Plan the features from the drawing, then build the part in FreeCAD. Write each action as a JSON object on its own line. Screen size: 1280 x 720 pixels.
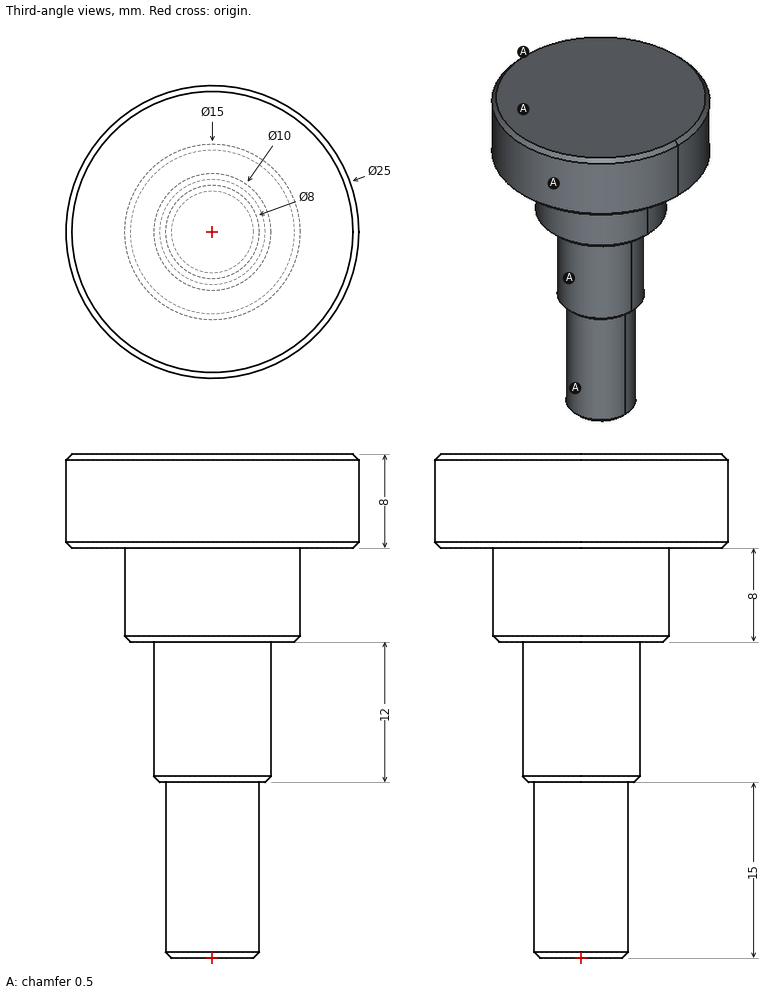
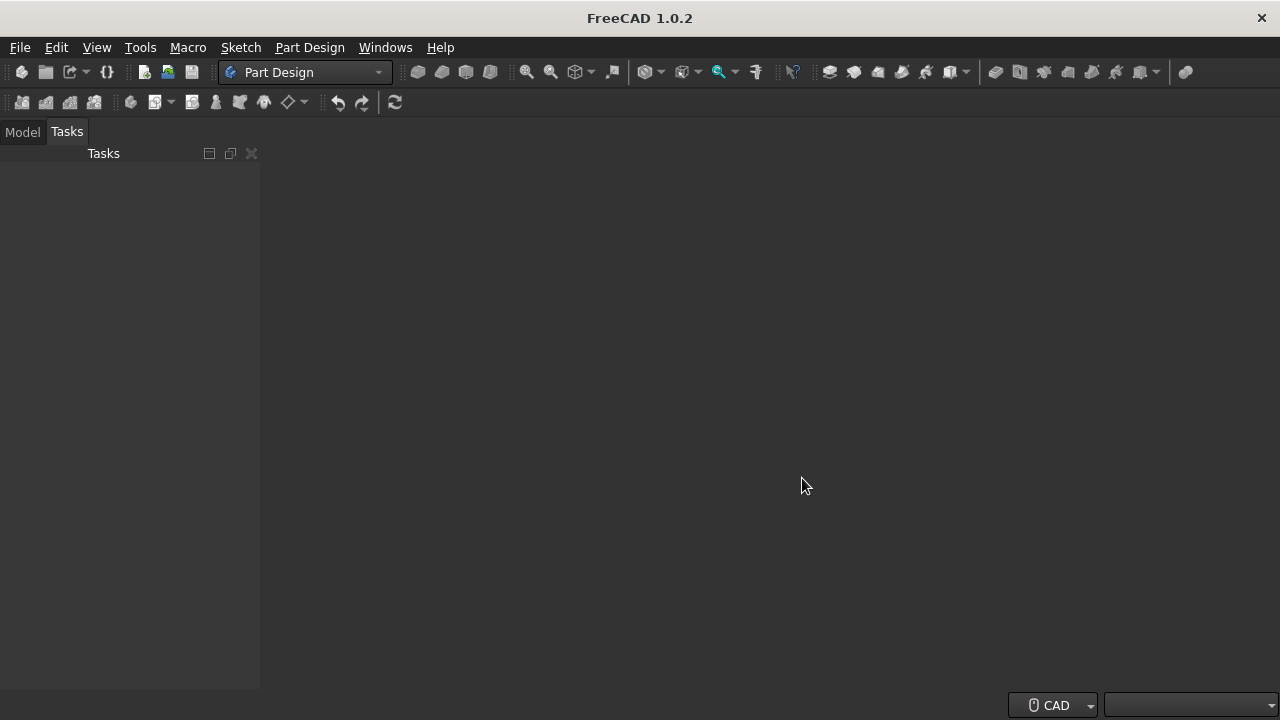
{"action": "left_click", "coordinate": [144, 72]}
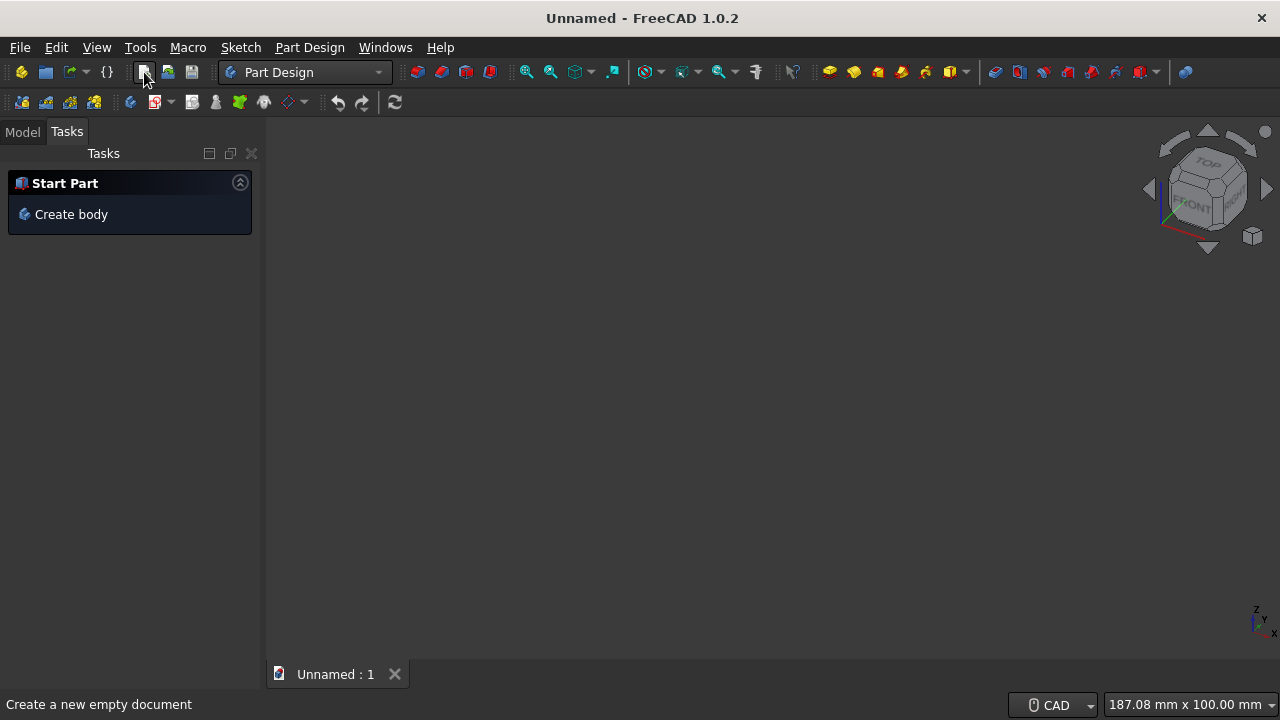
{"action": "left_click", "coordinate": [156, 102]}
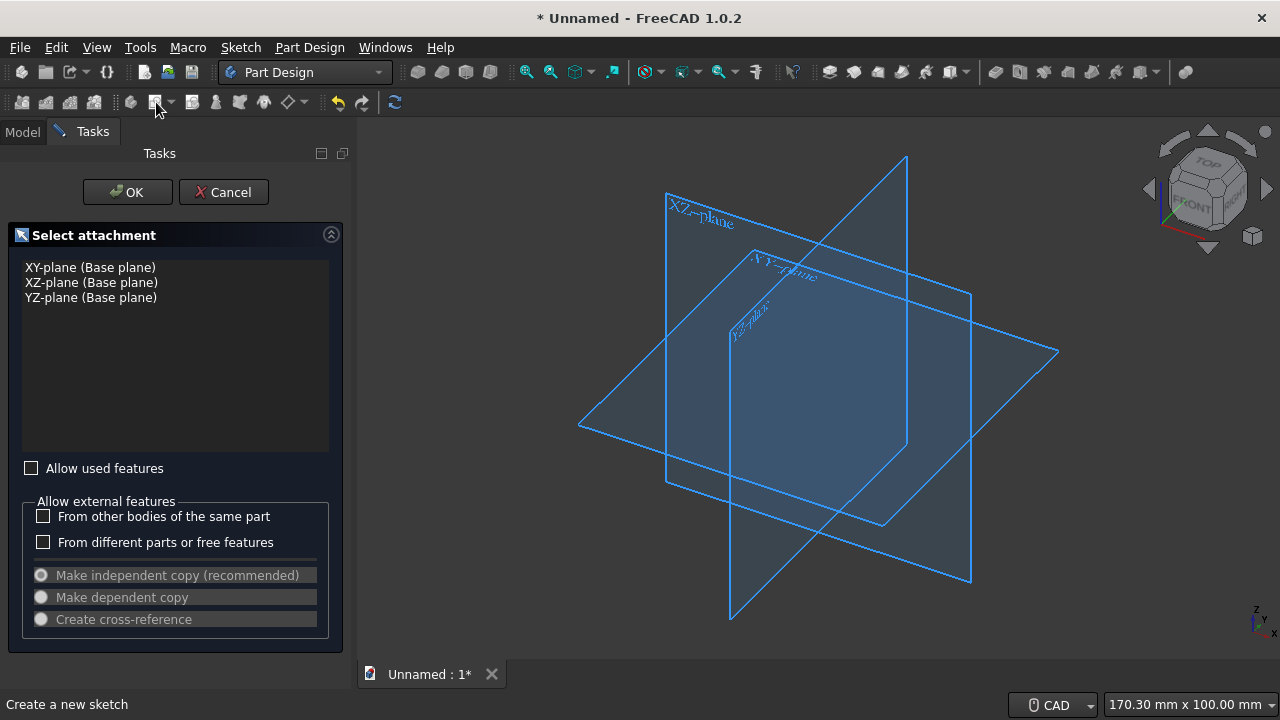
{"action": "left_click", "coordinate": [82, 268]}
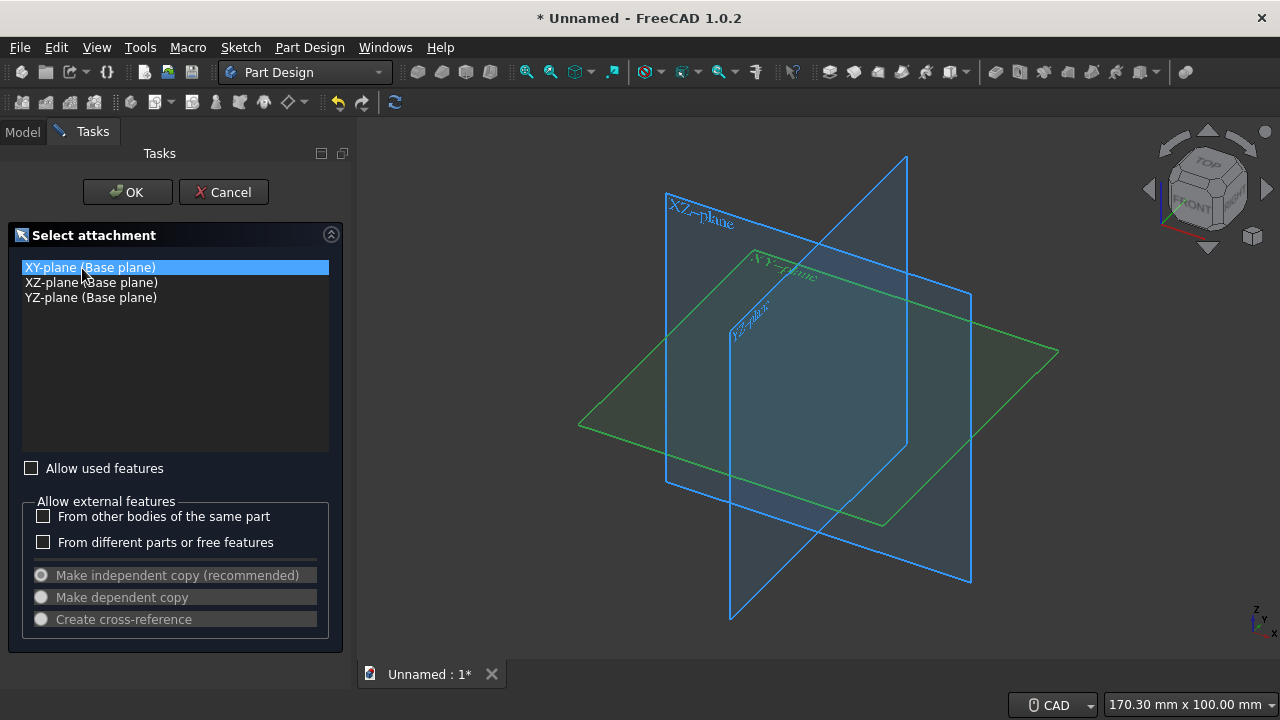
{"action": "left_click", "coordinate": [128, 192]}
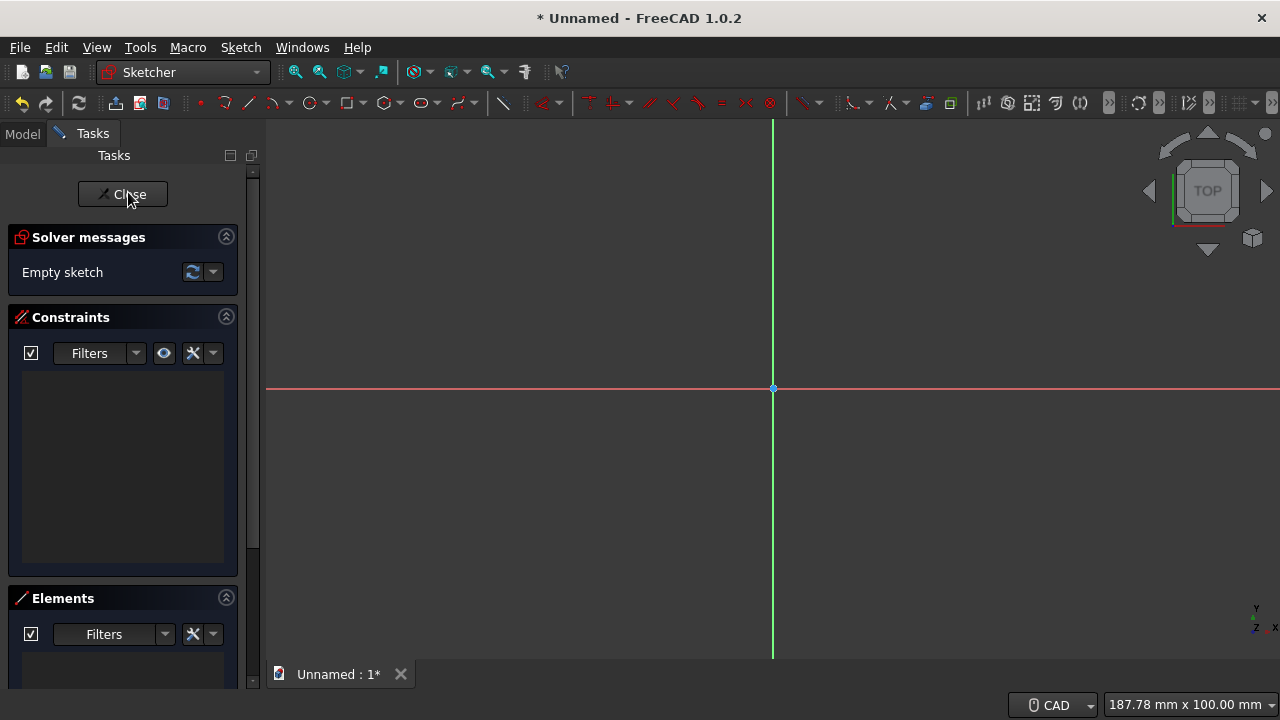
{"action": "scroll", "coordinate": [784, 389], "scroll_direction": "up", "scroll_amount": 10}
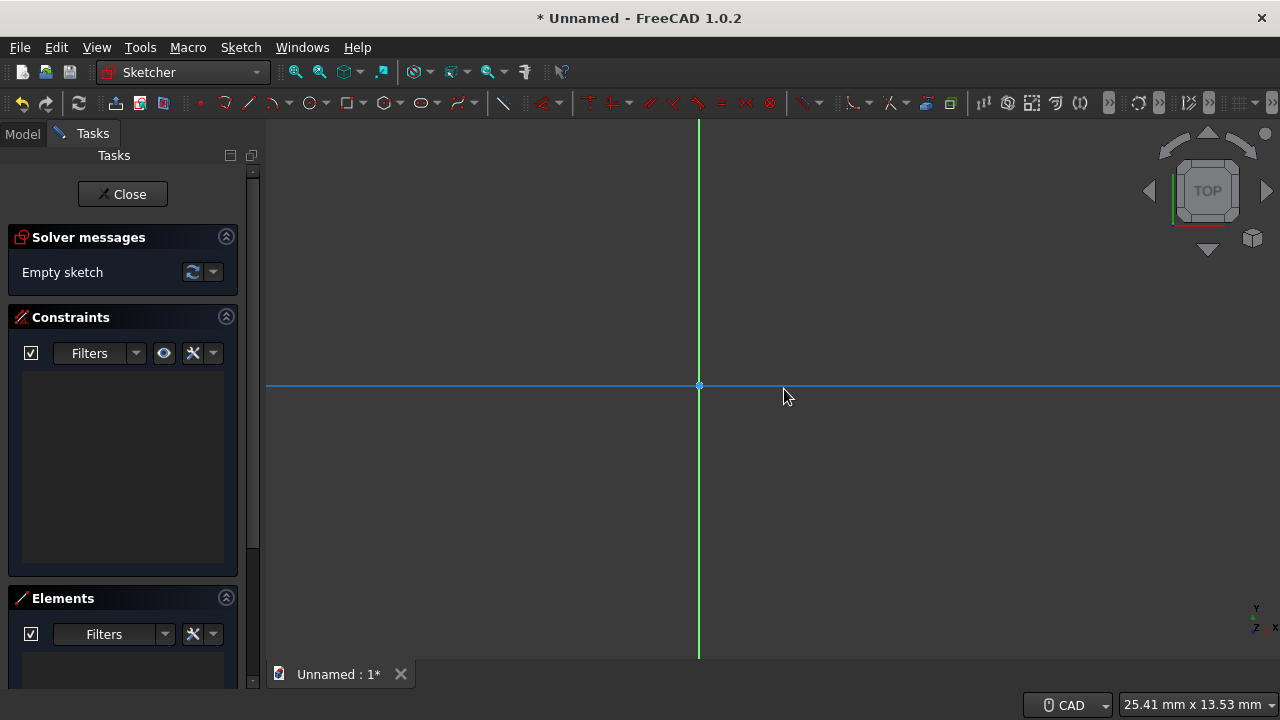
{"action": "left_click", "coordinate": [310, 104]}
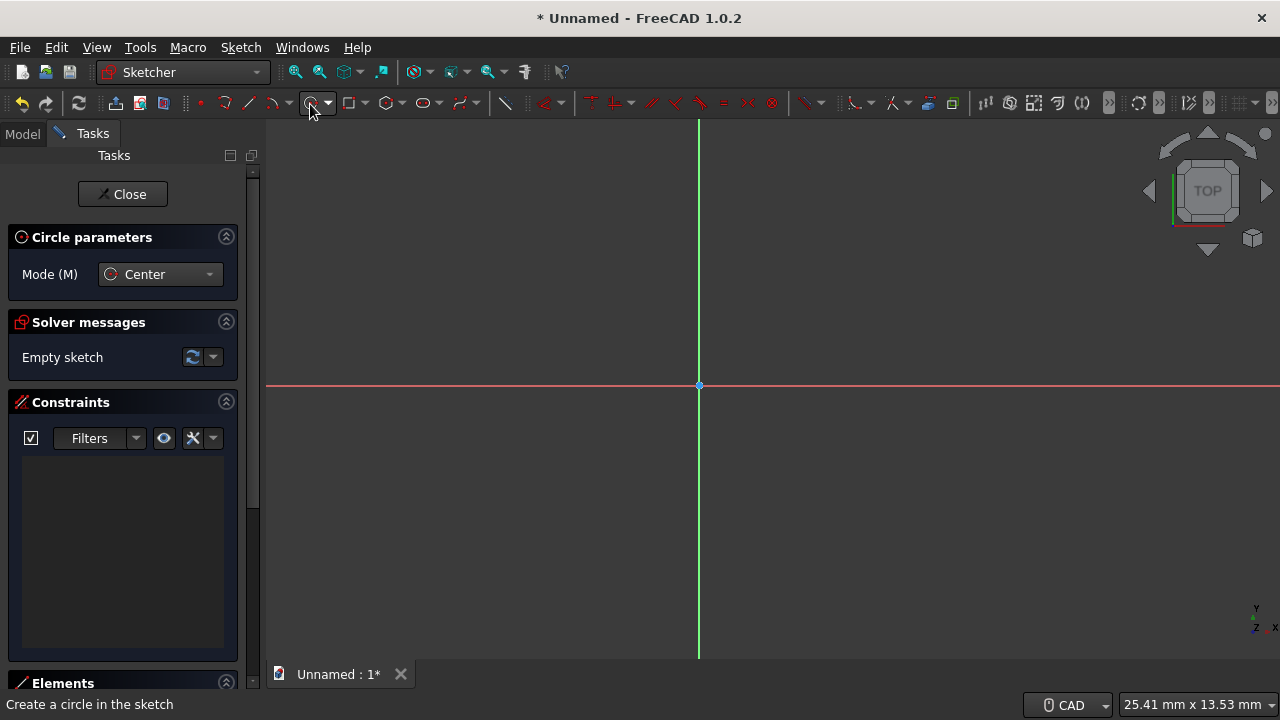
{"action": "left_click", "coordinate": [699, 386]}
{"action": "left_click", "coordinate": [812, 273]}
{"action": "key", "text": "Escape"}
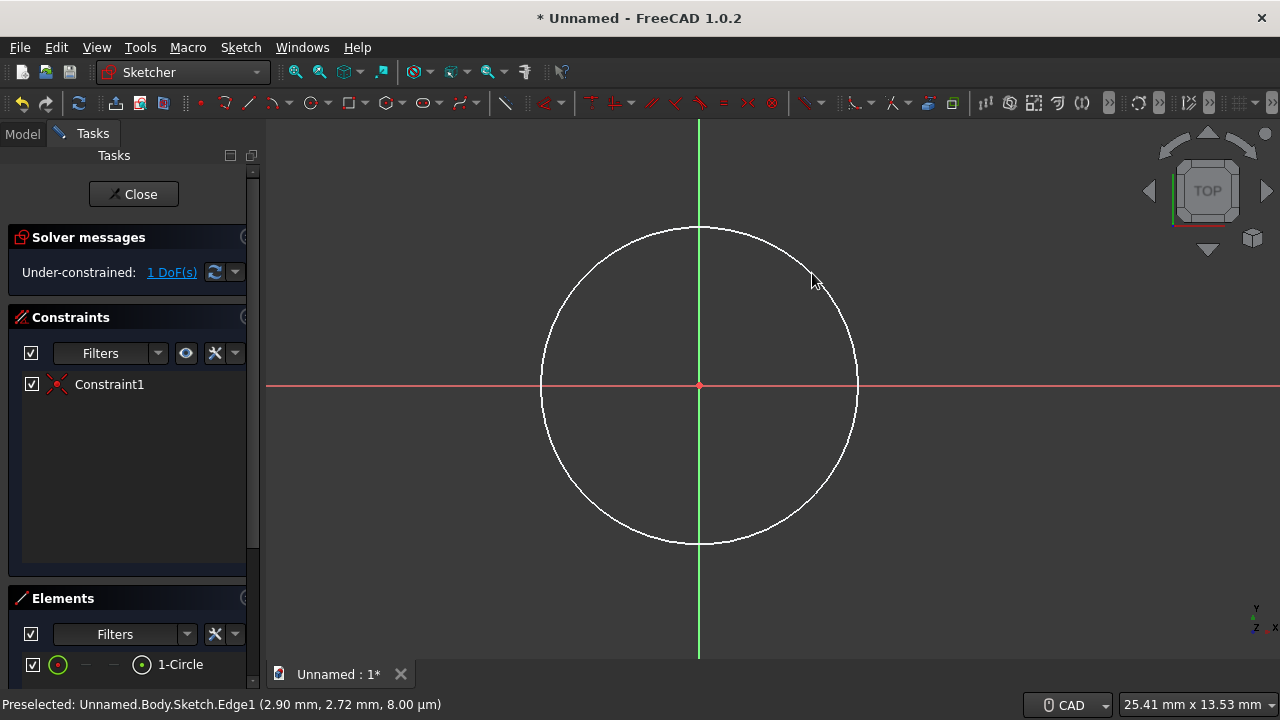
{"action": "left_click", "coordinate": [544, 104]}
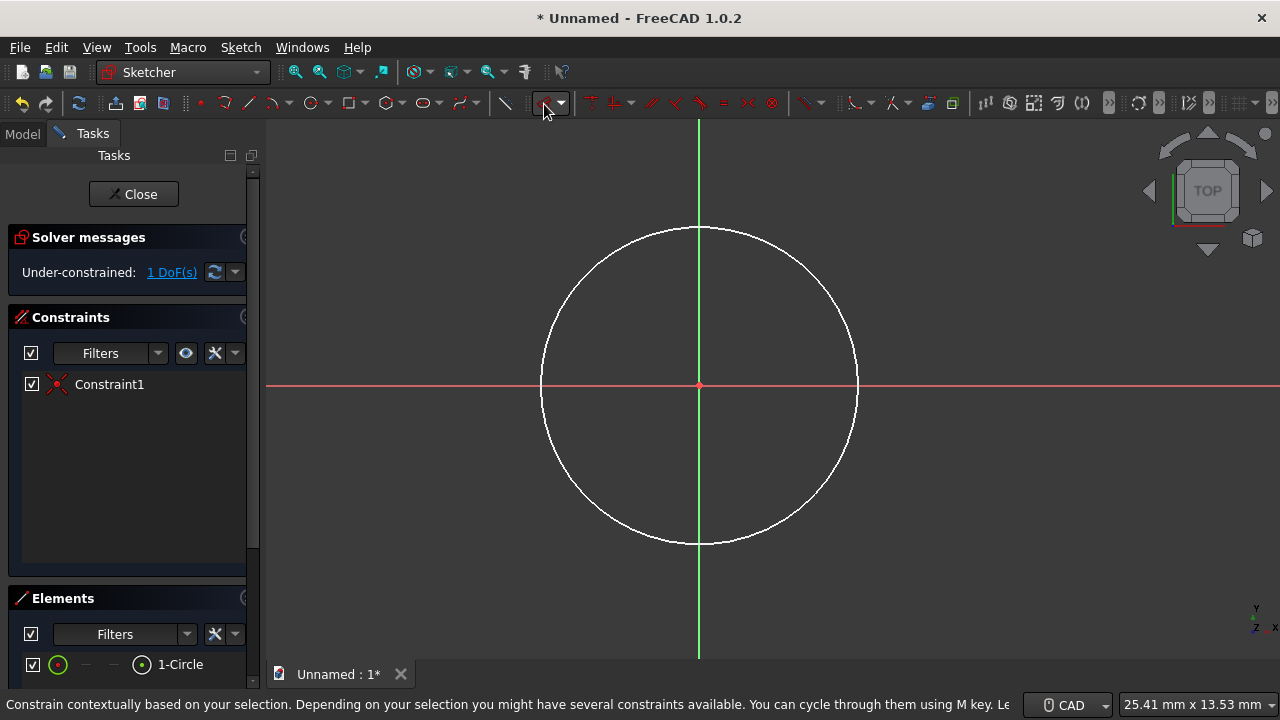
{"action": "left_click", "coordinate": [811, 273]}
{"action": "left_click", "coordinate": [834, 250]}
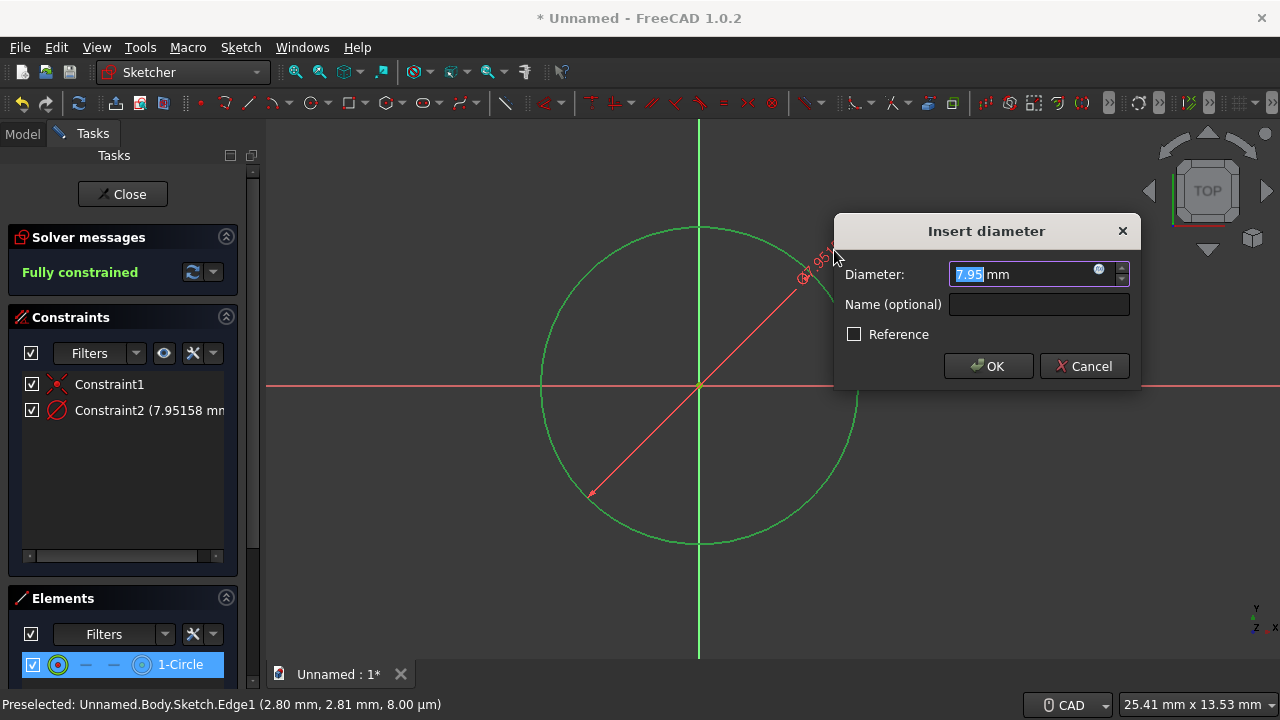
{"action": "type", "text": "8"}
{"action": "key", "text": "Return"}
{"action": "key", "text": "Escape"}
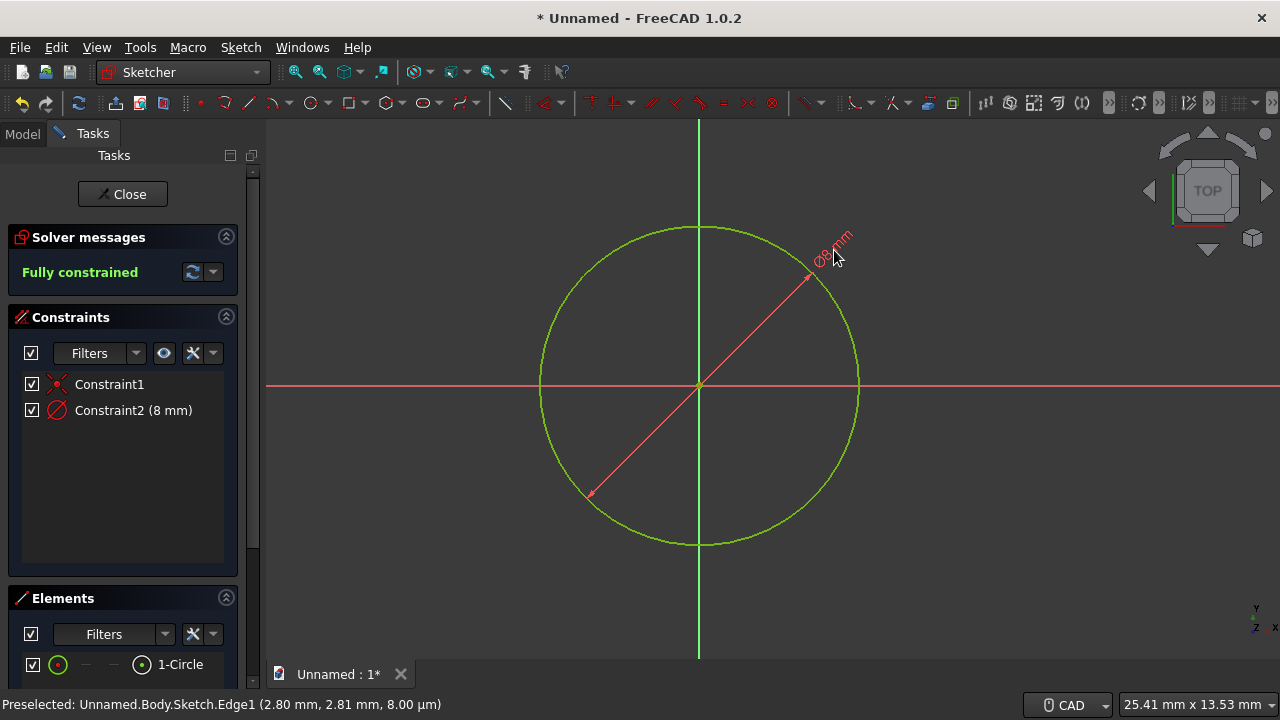
{"action": "left_click", "coordinate": [123, 194]}